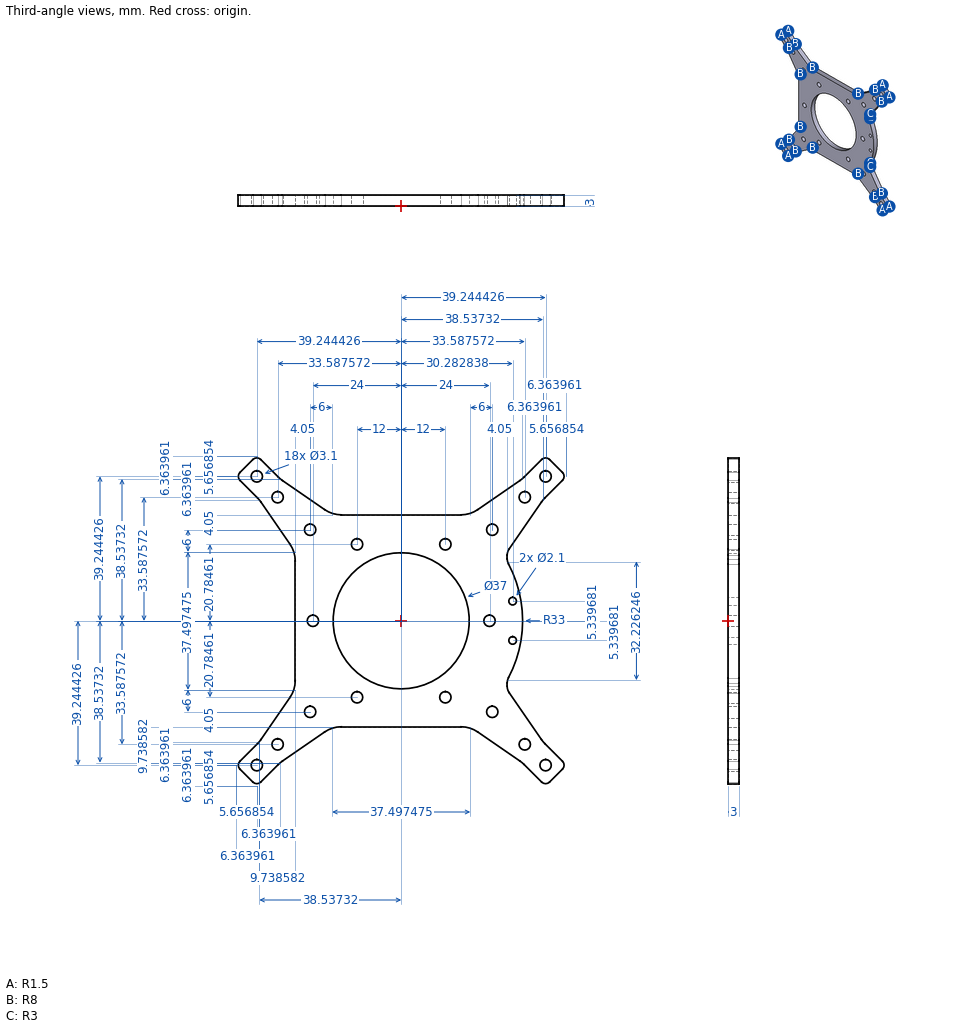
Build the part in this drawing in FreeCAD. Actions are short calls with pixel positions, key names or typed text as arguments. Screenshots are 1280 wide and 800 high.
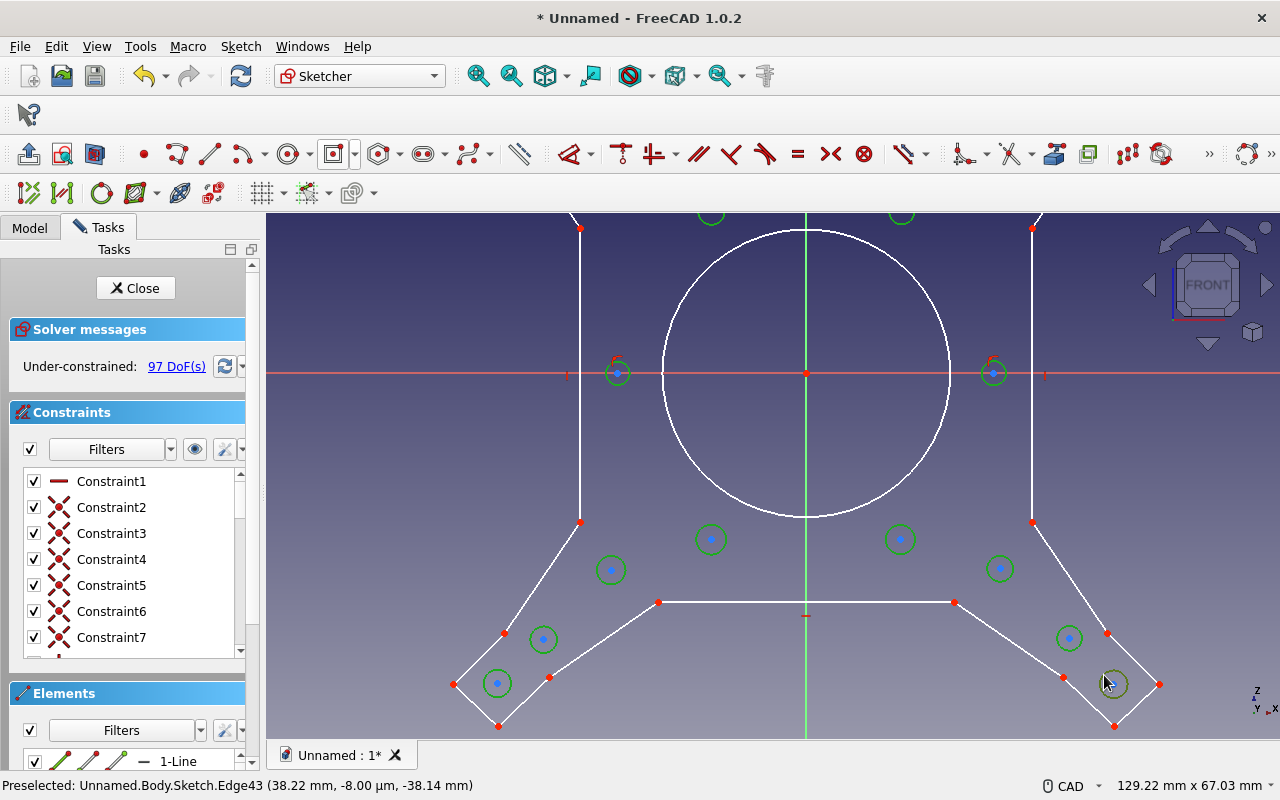
click(798, 154)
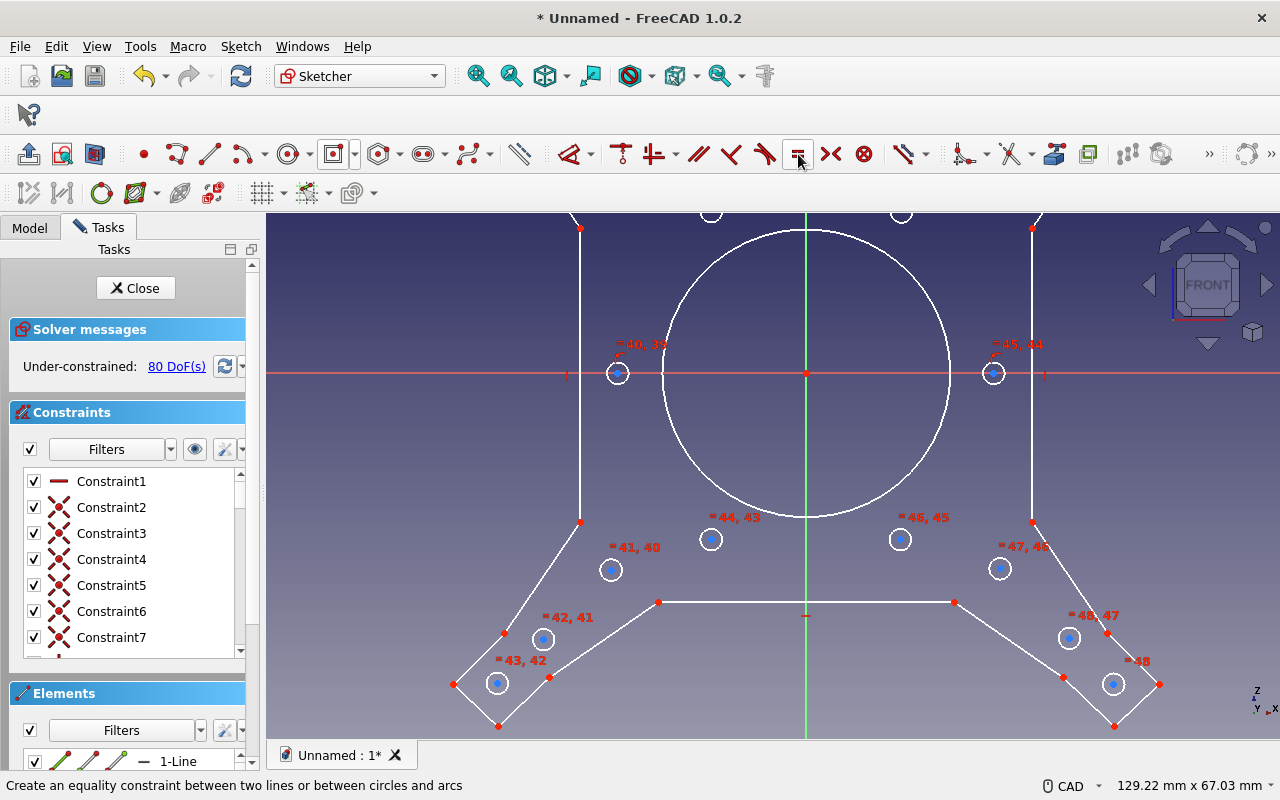
scroll(621, 560, down, 4)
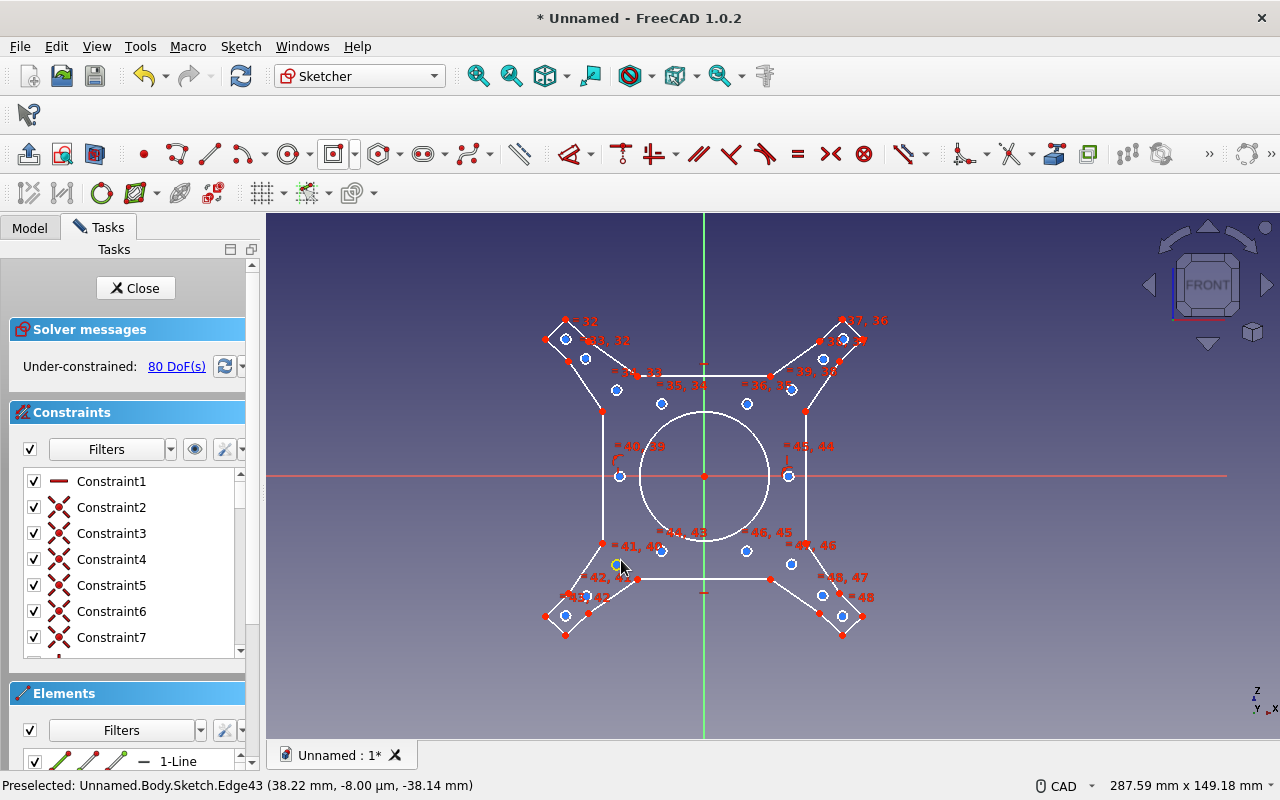
click(662, 404)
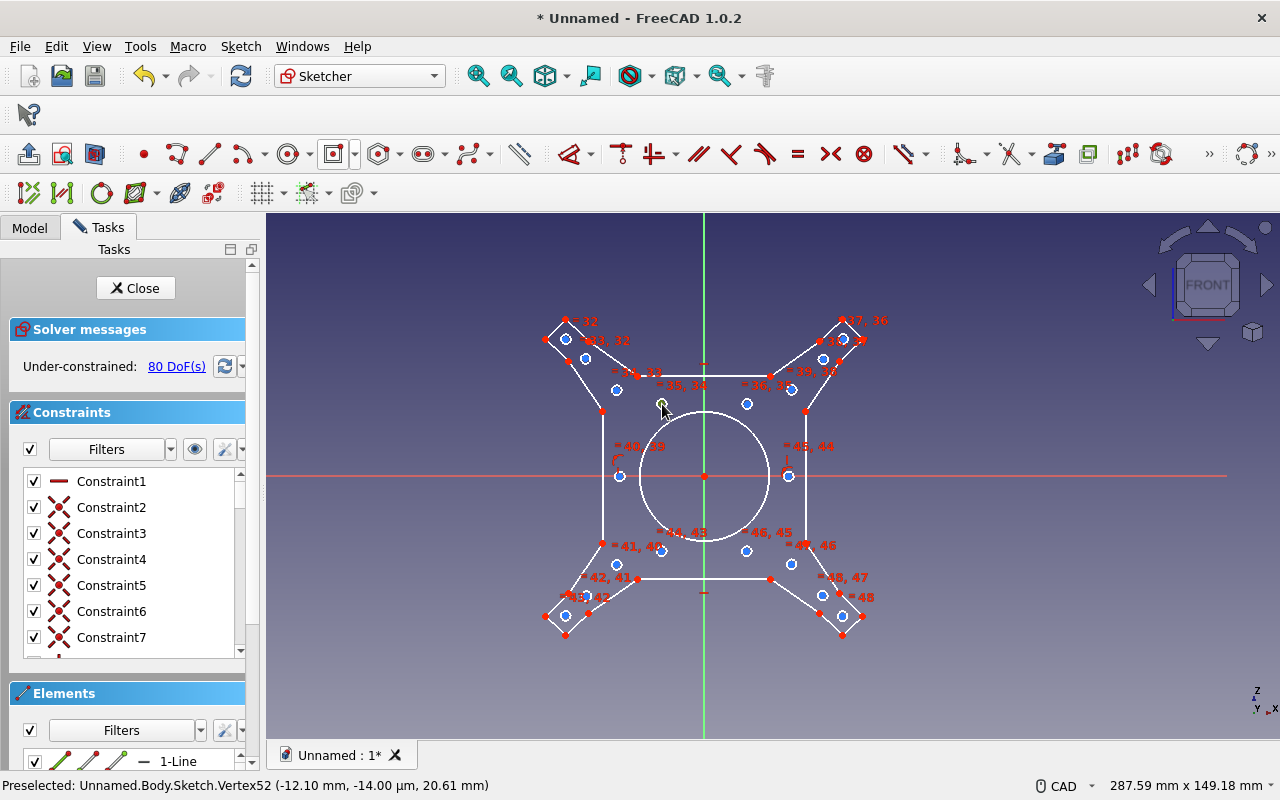
click(747, 404)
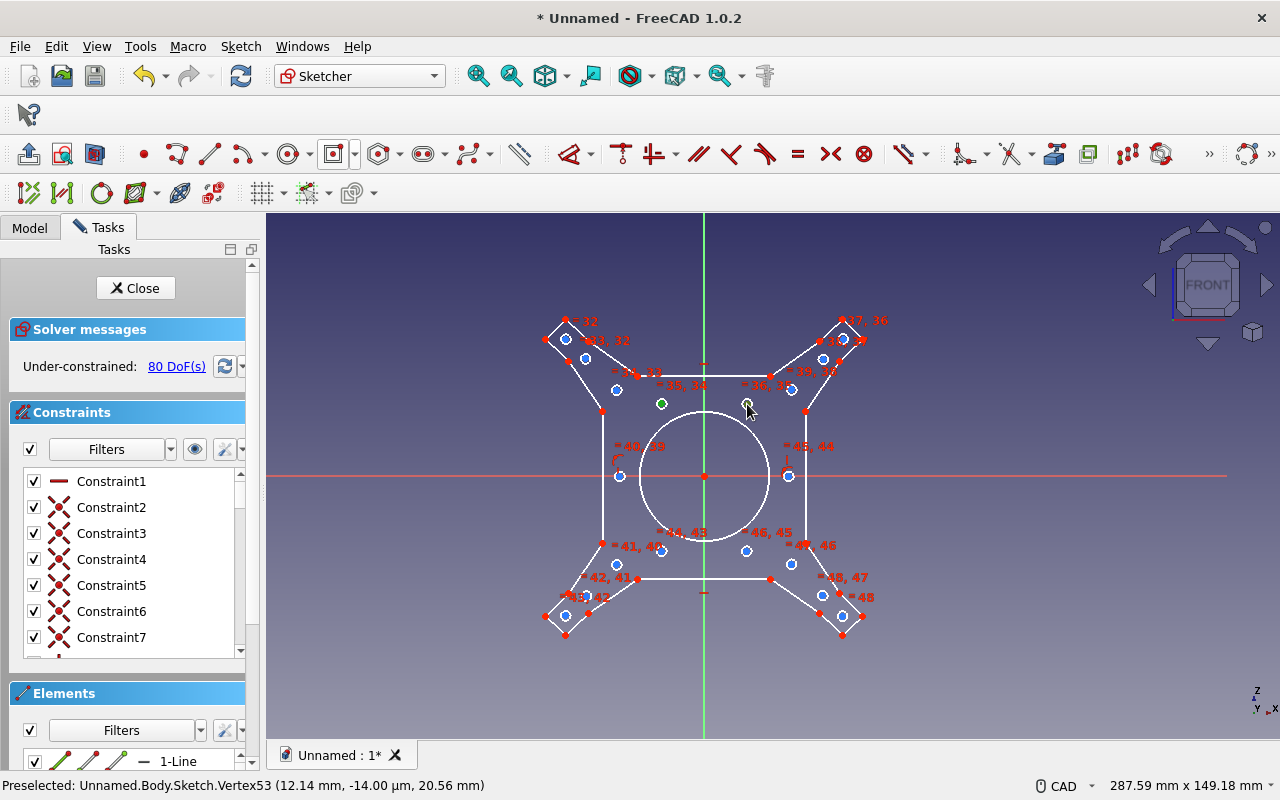
key(h)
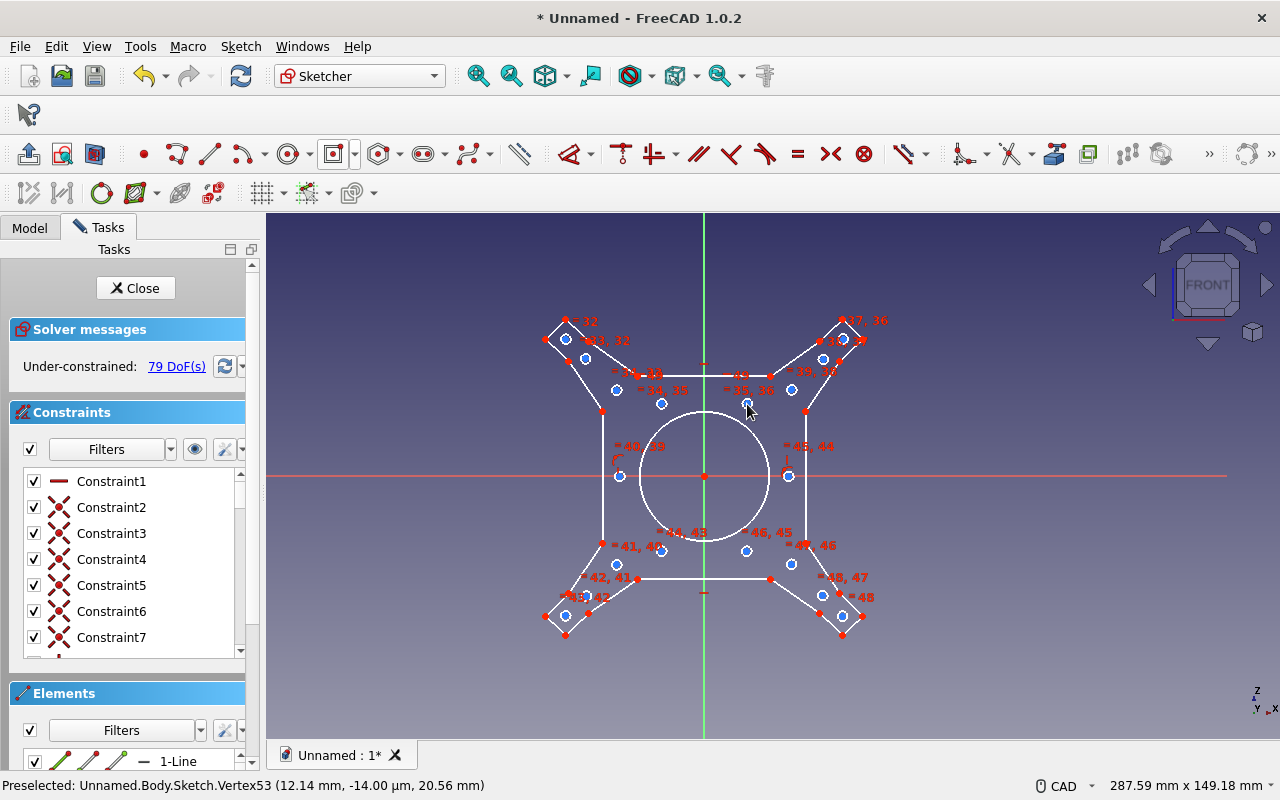
click(662, 551)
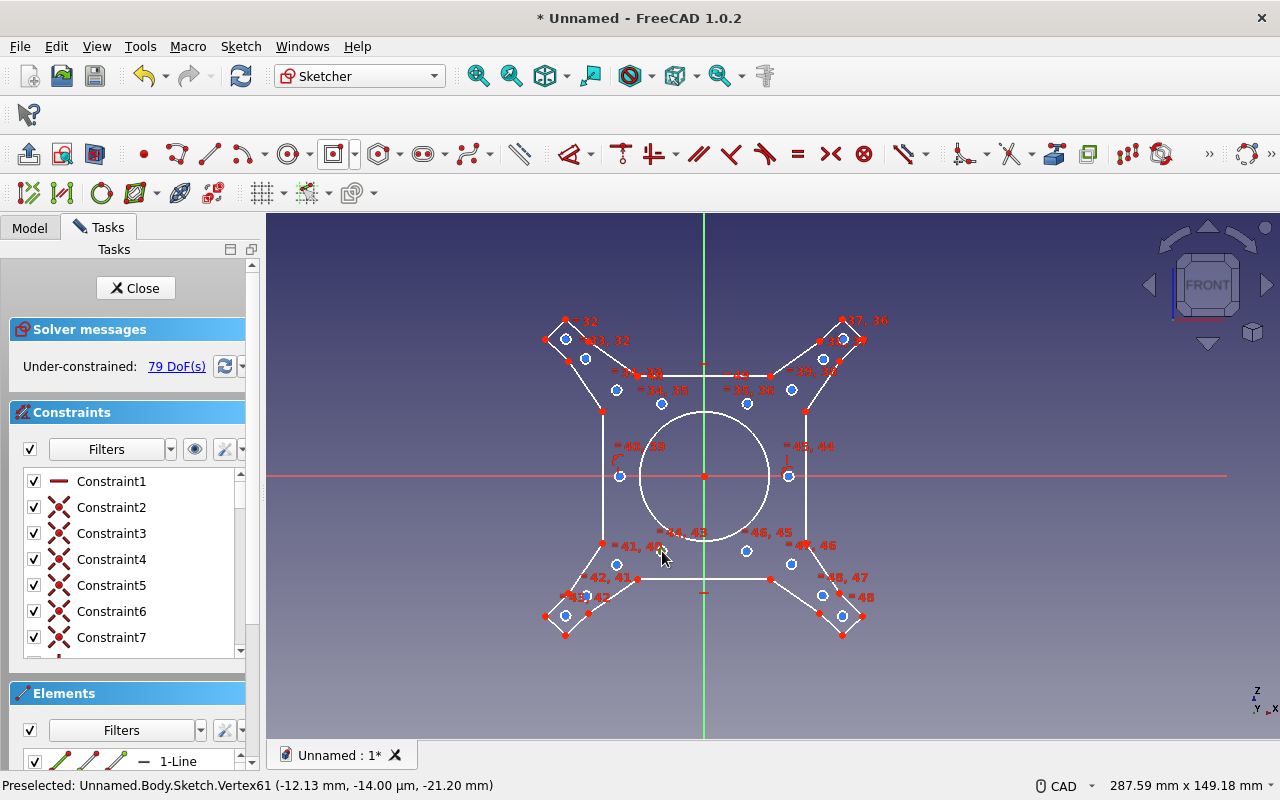
click(747, 551)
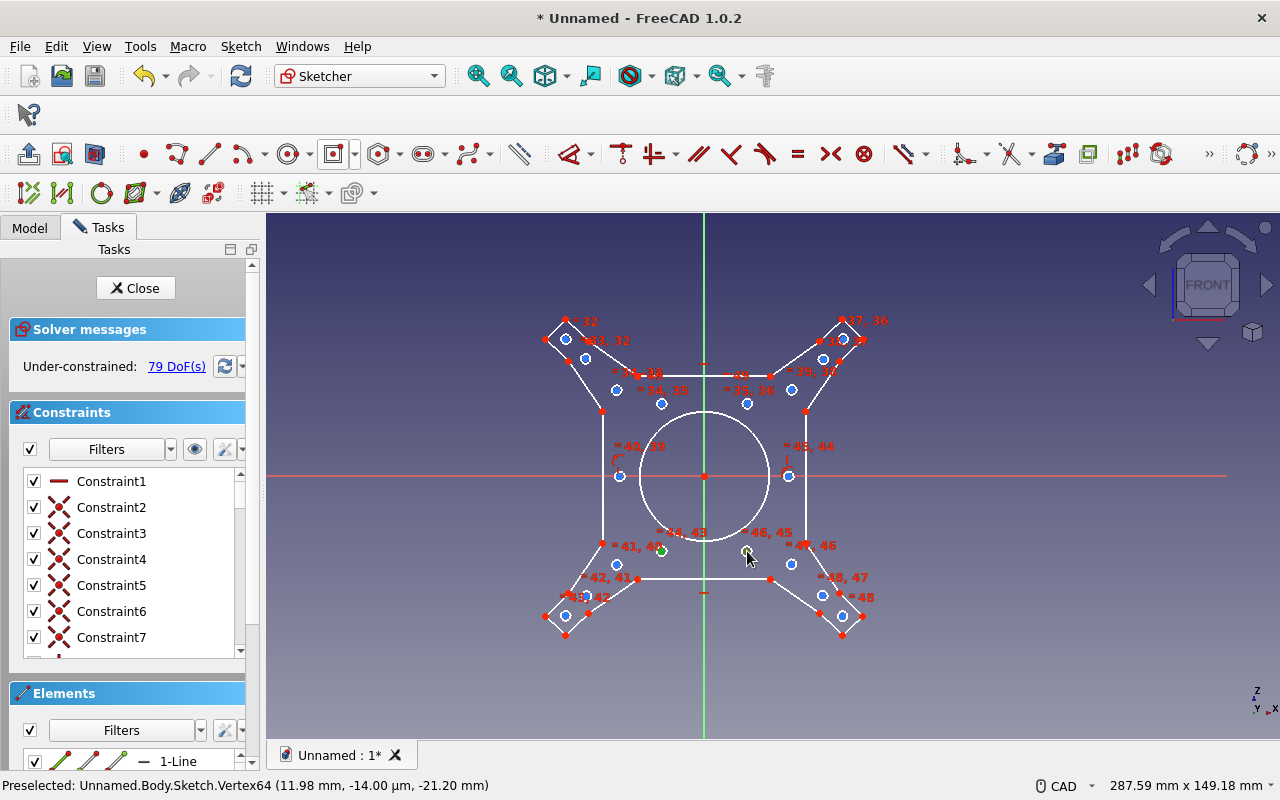
click(676, 154)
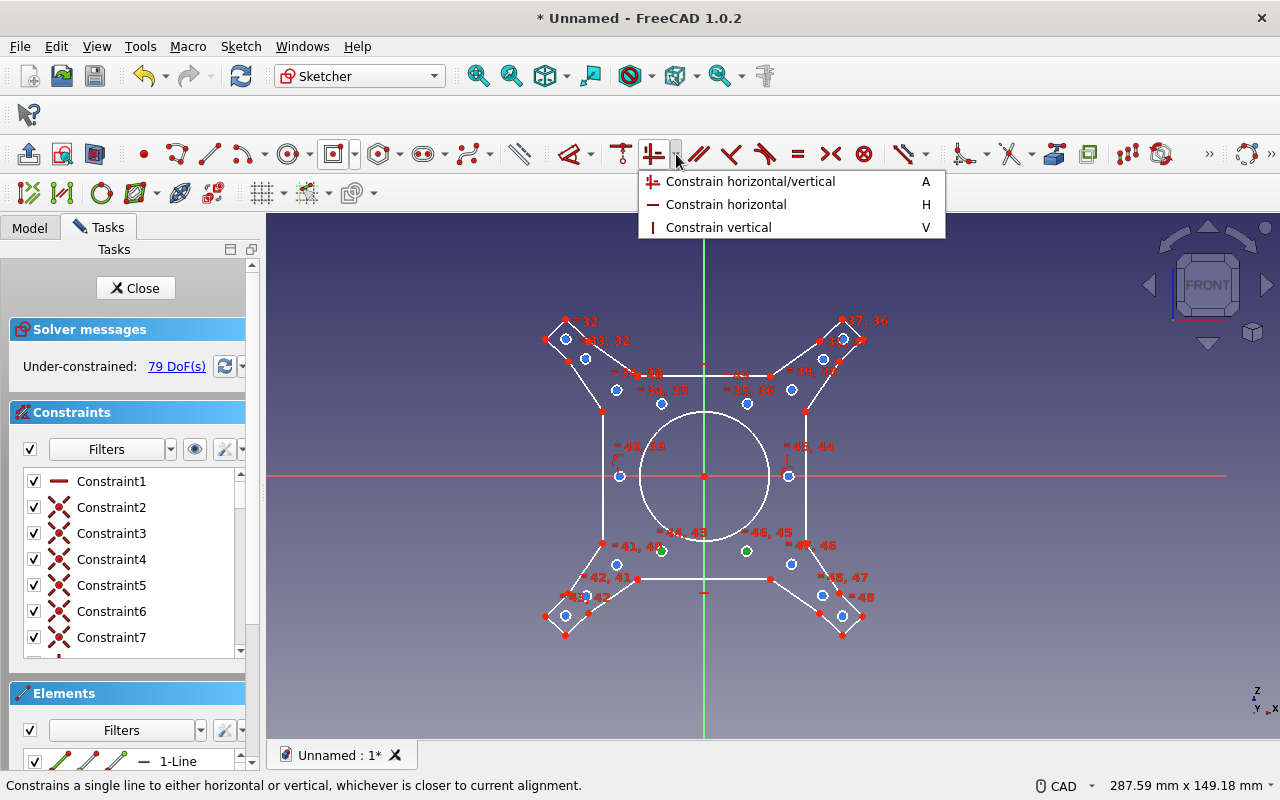
click(792, 204)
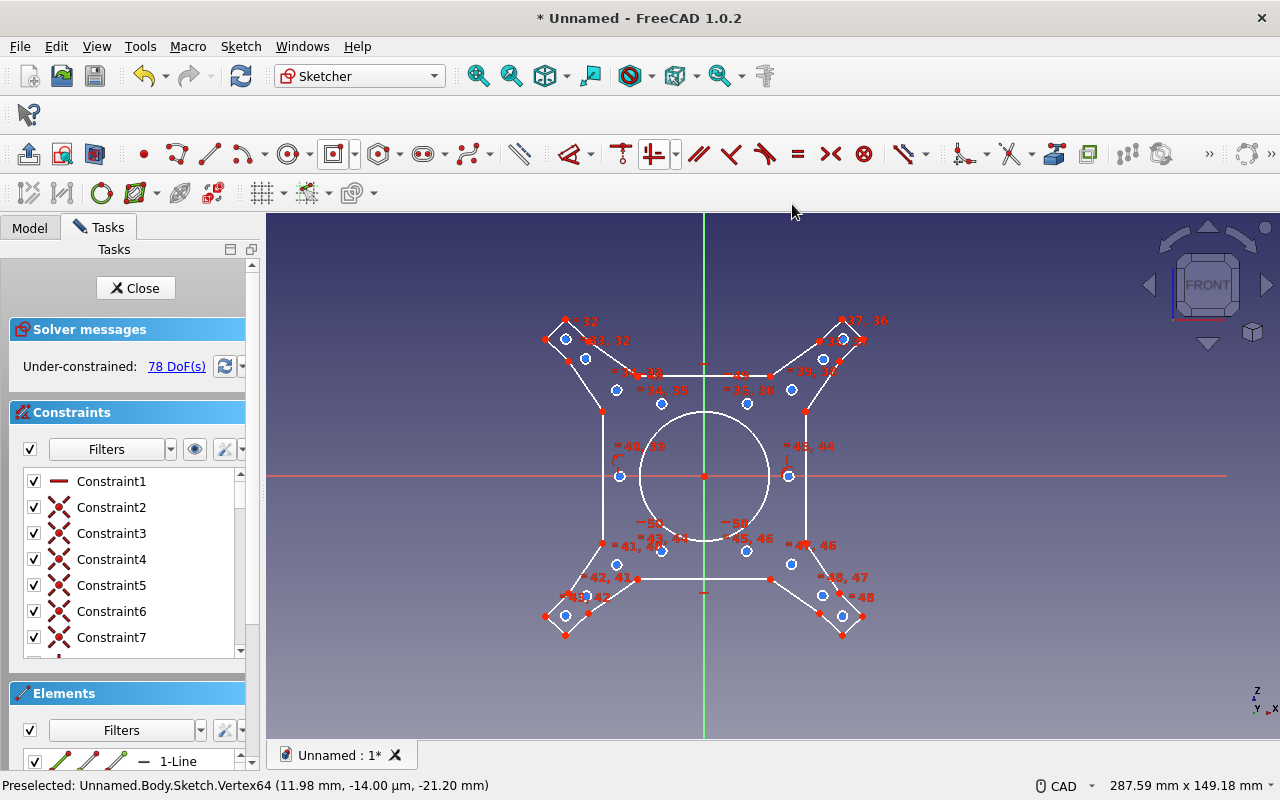
key(d)